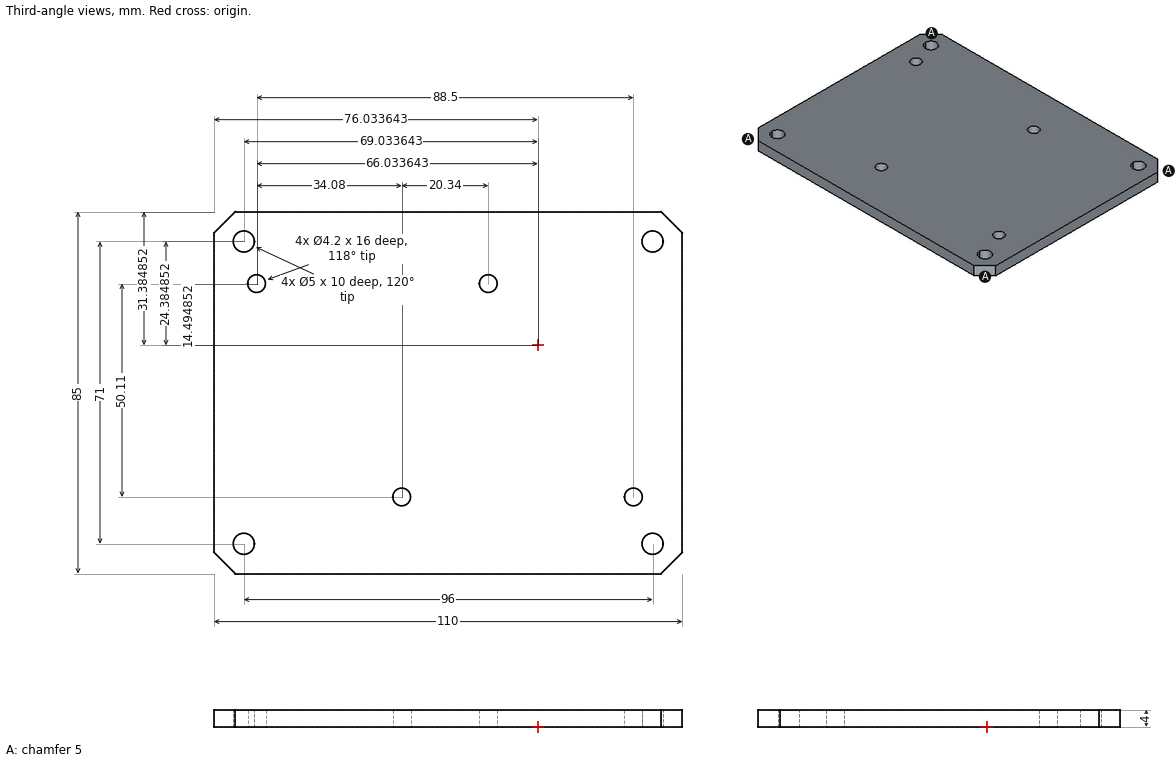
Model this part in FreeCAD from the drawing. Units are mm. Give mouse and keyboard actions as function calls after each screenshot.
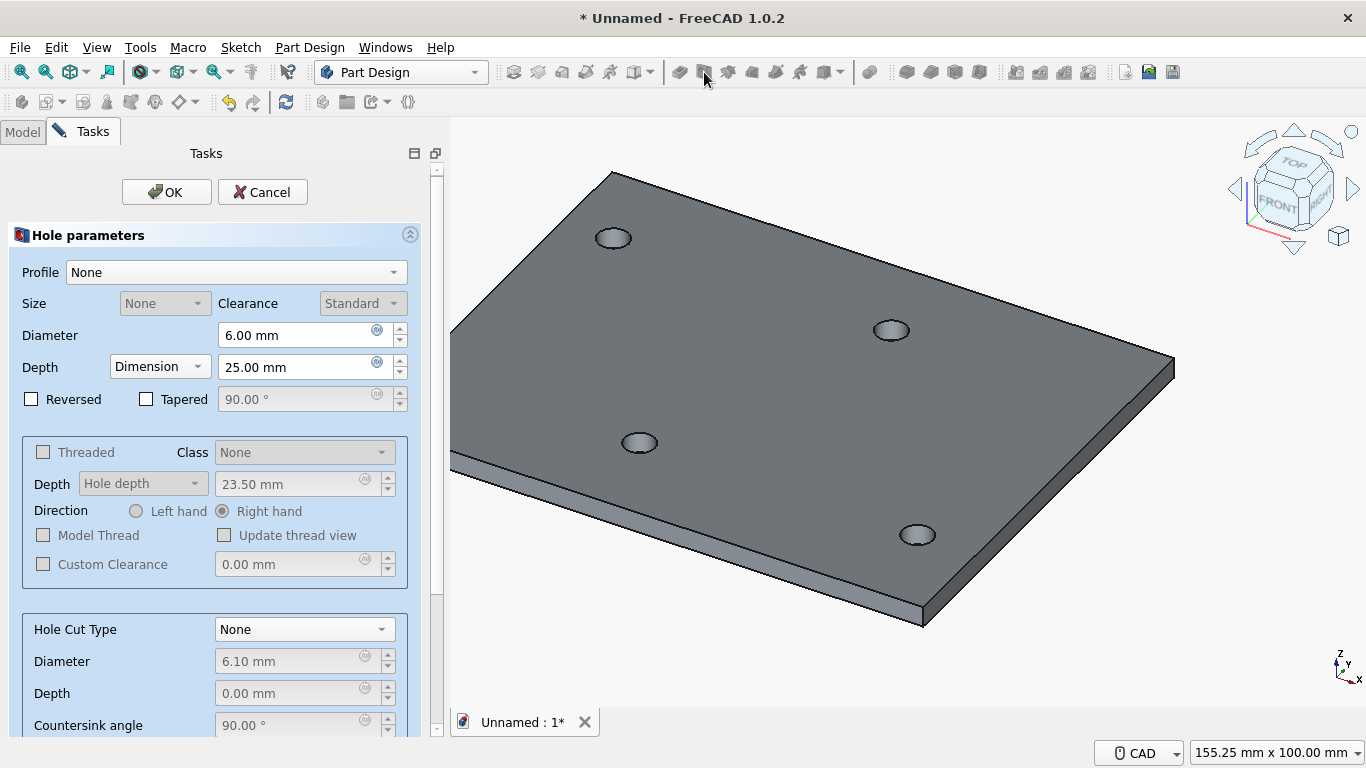
triple_click(305, 335)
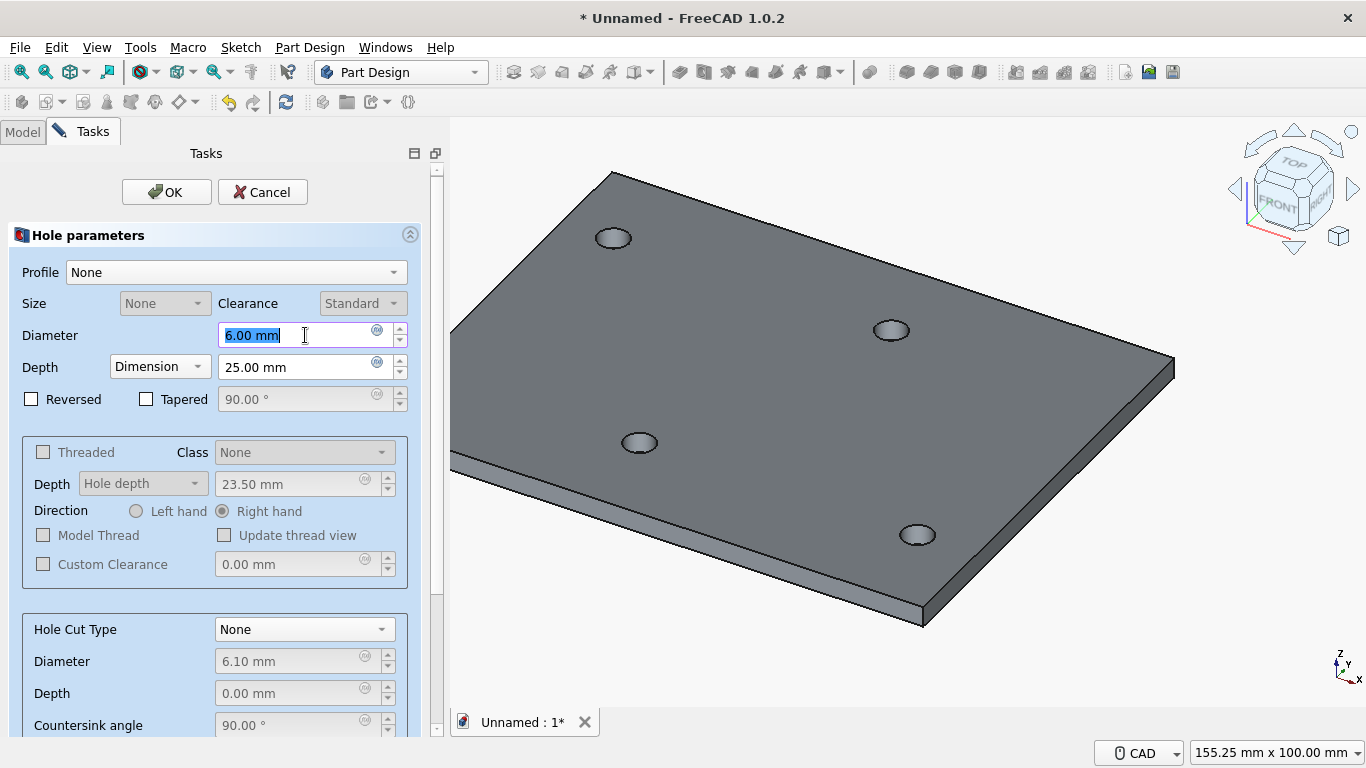
text(4.2)
key(Tab)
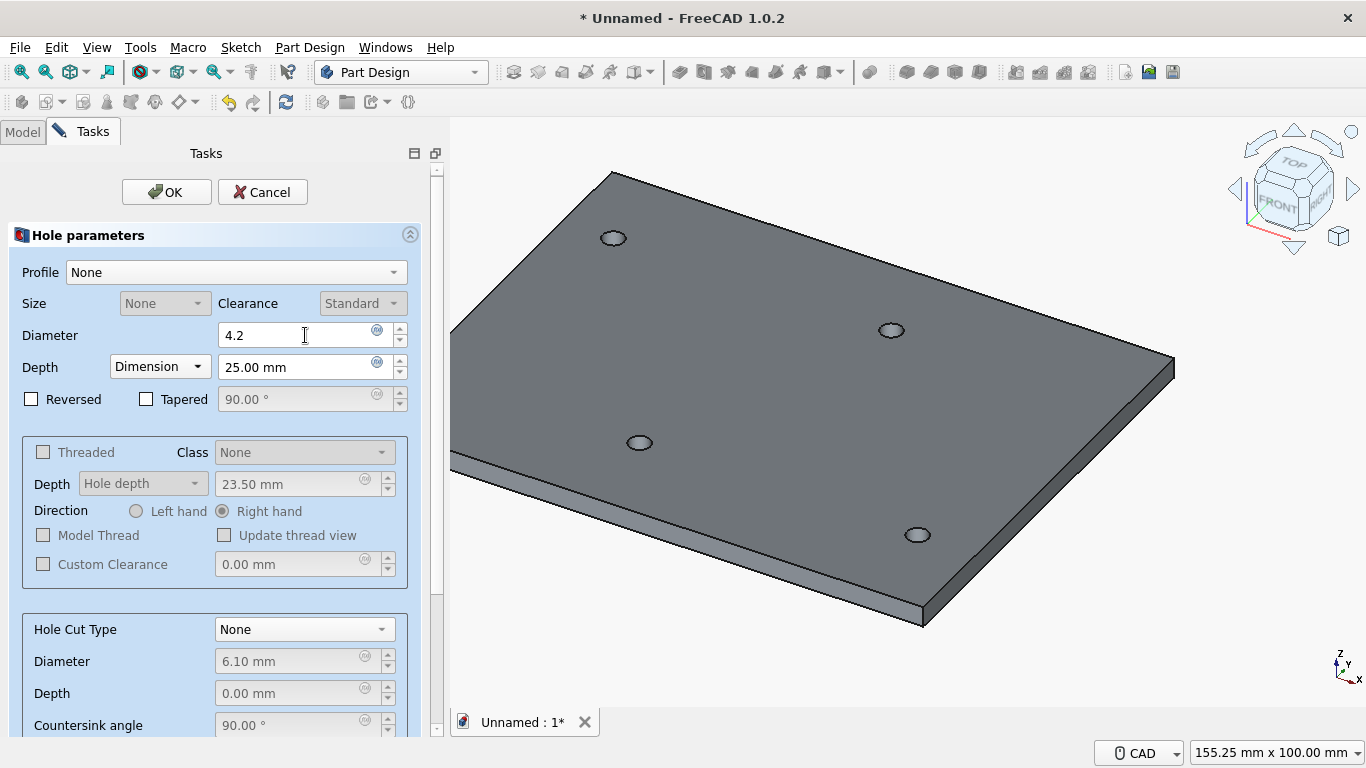
triple_click(305, 367)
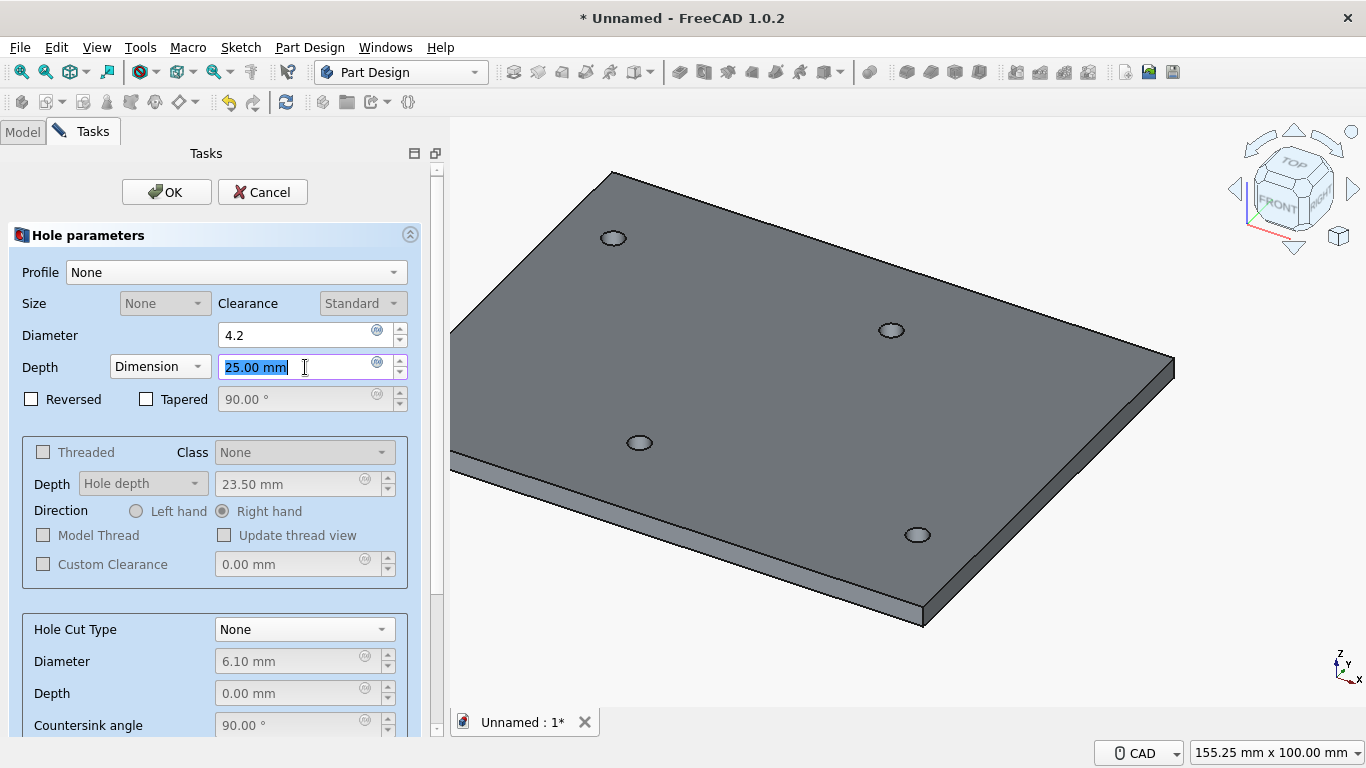
text(16)
key(Tab)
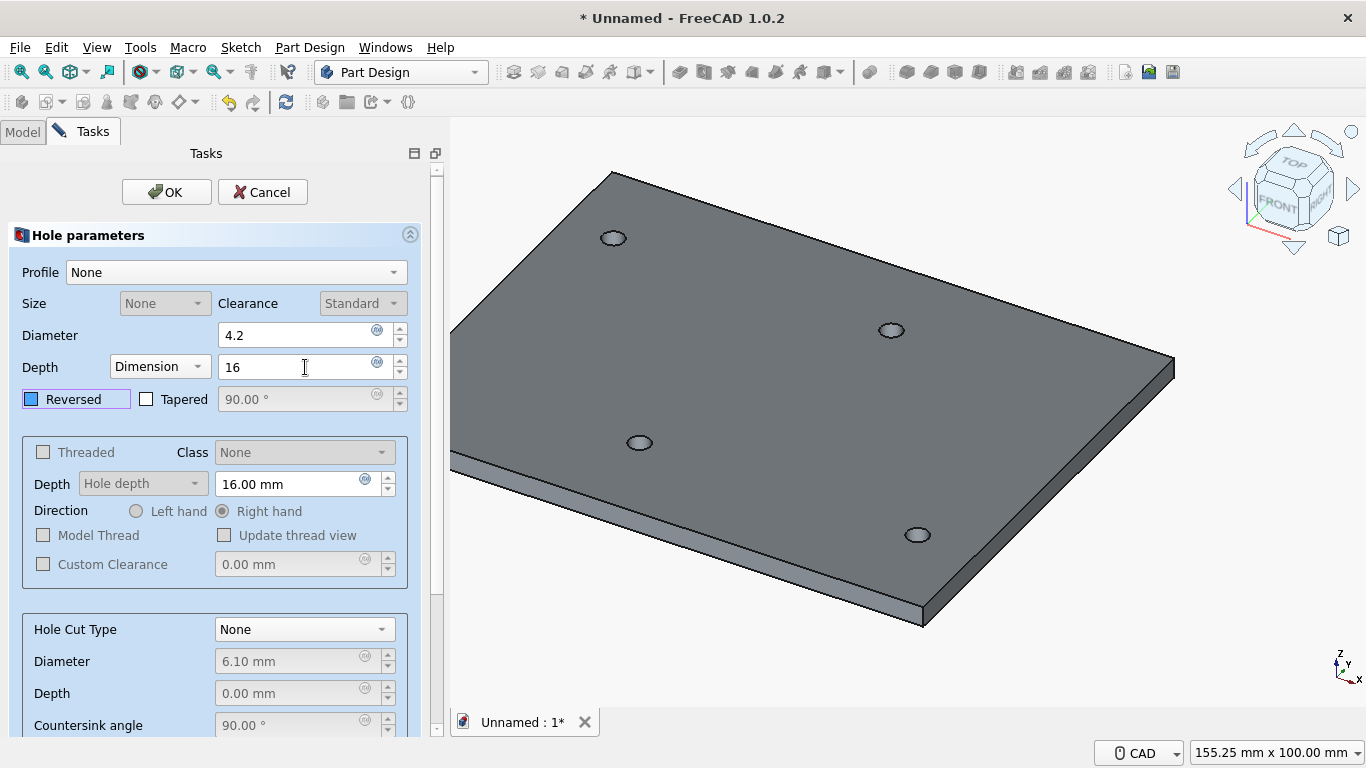
click(167, 192)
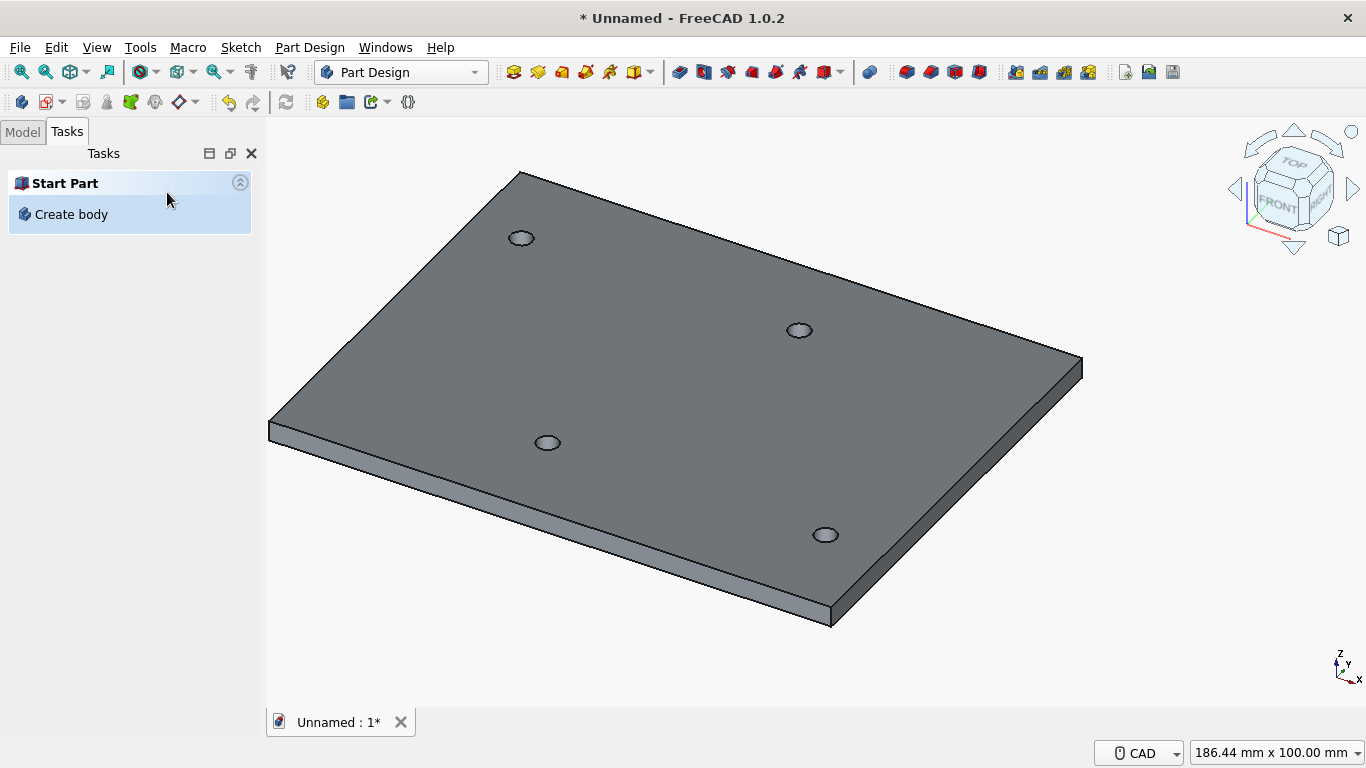
click(831, 616)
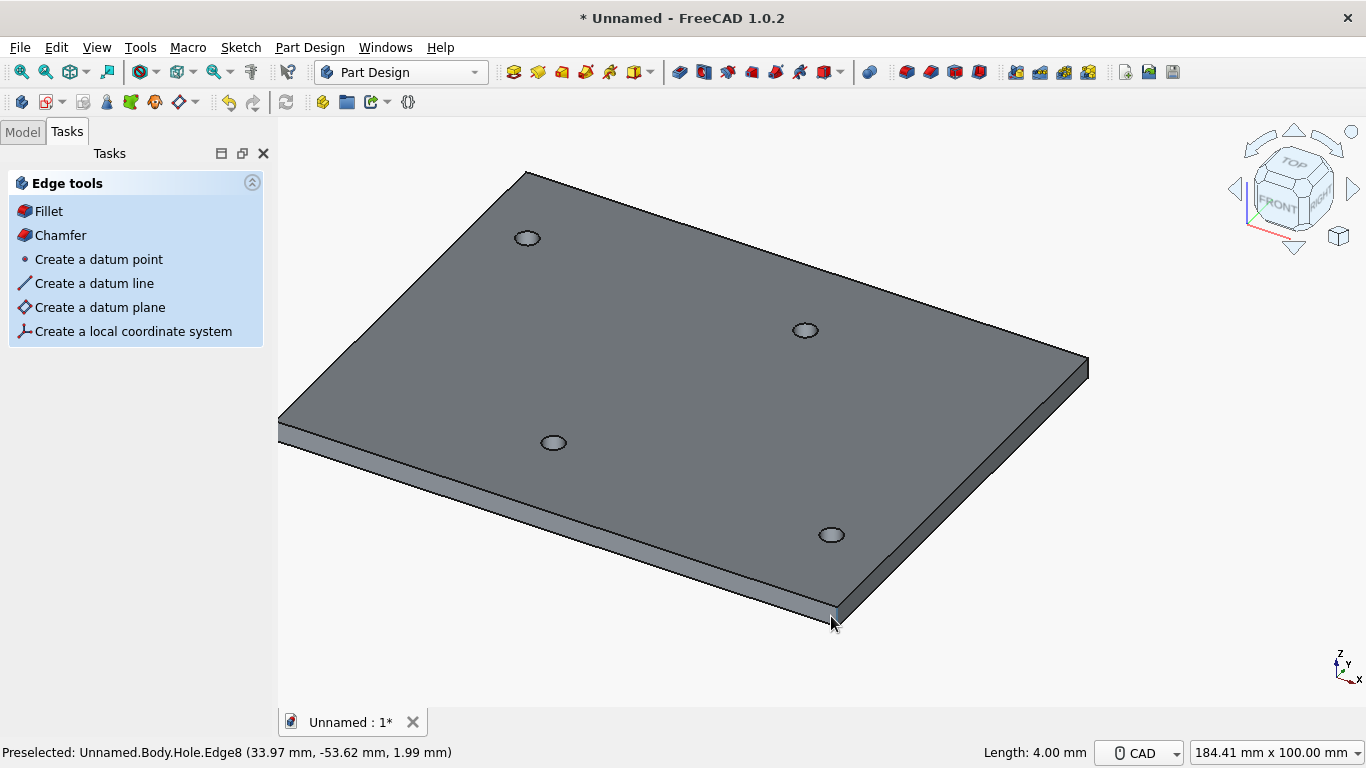
key(0)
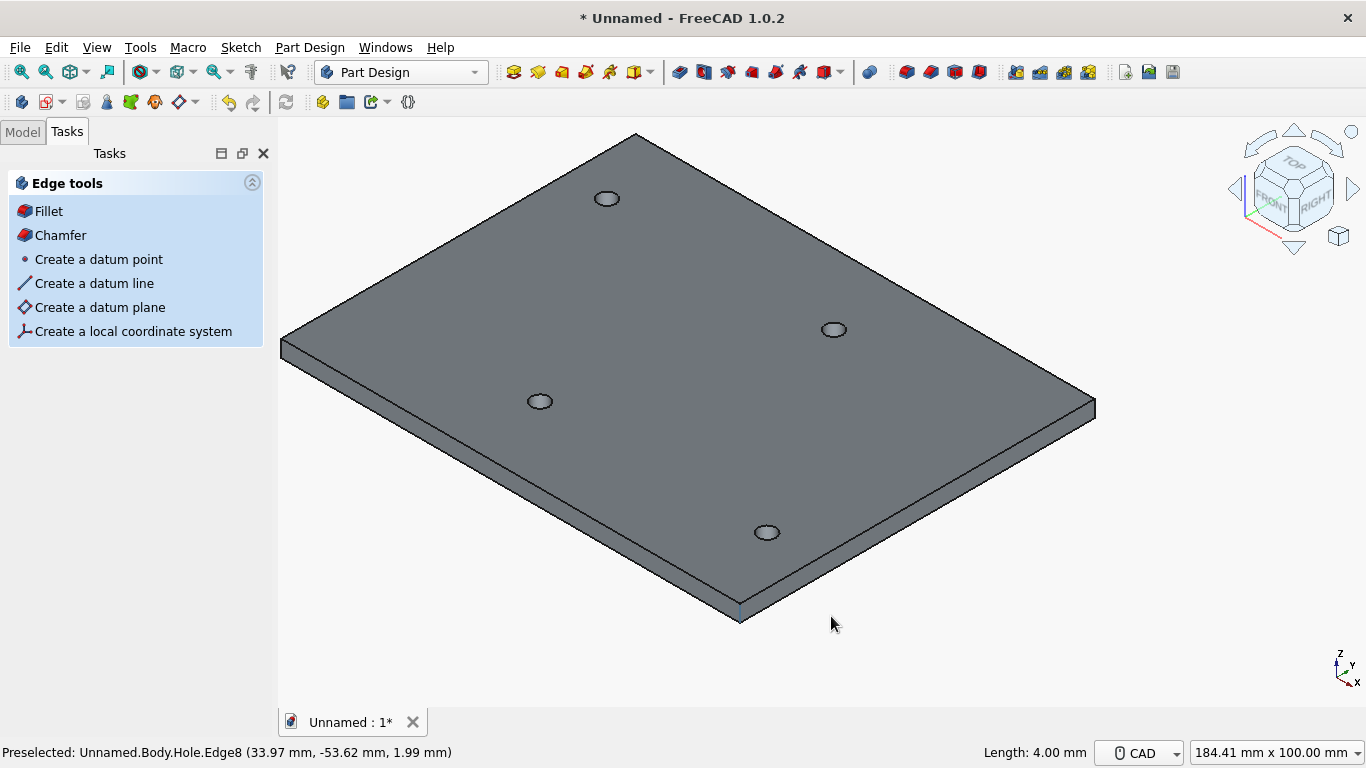
key(2)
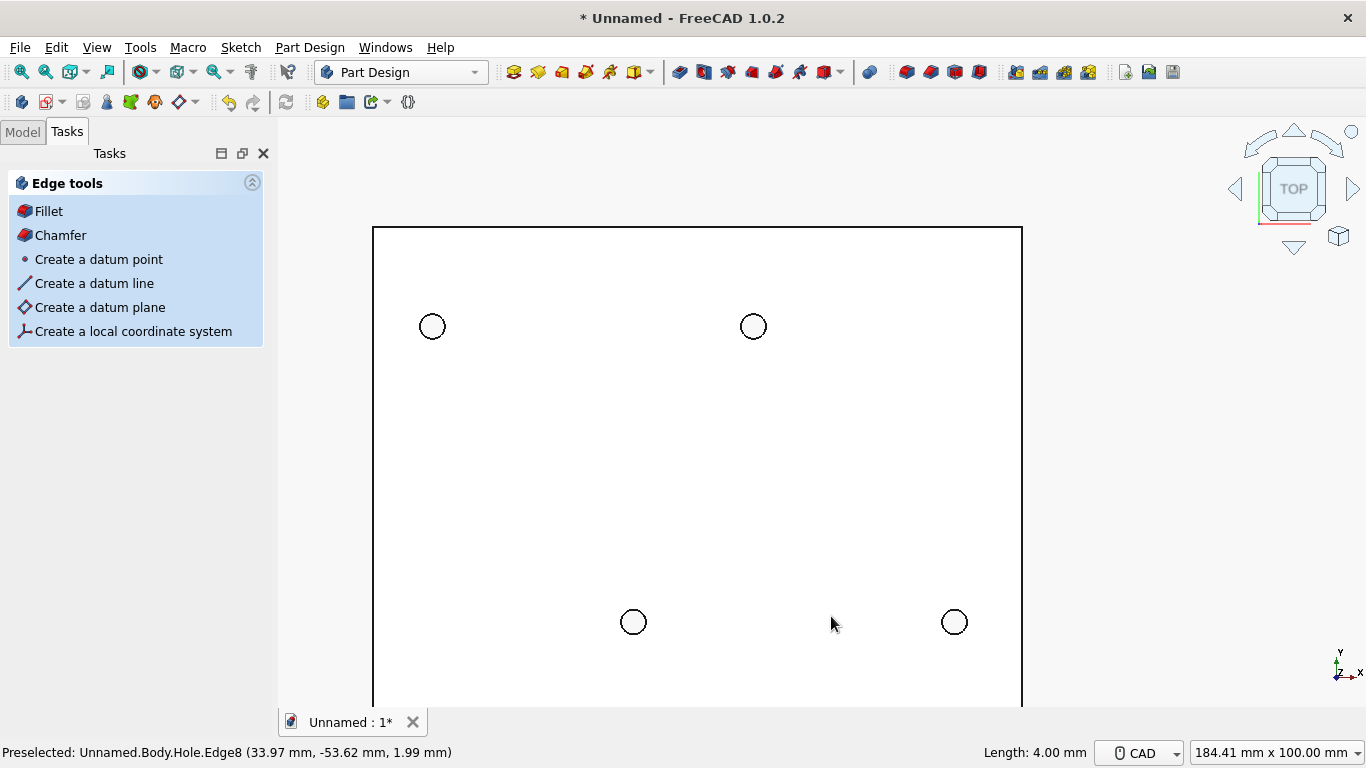
click(22, 72)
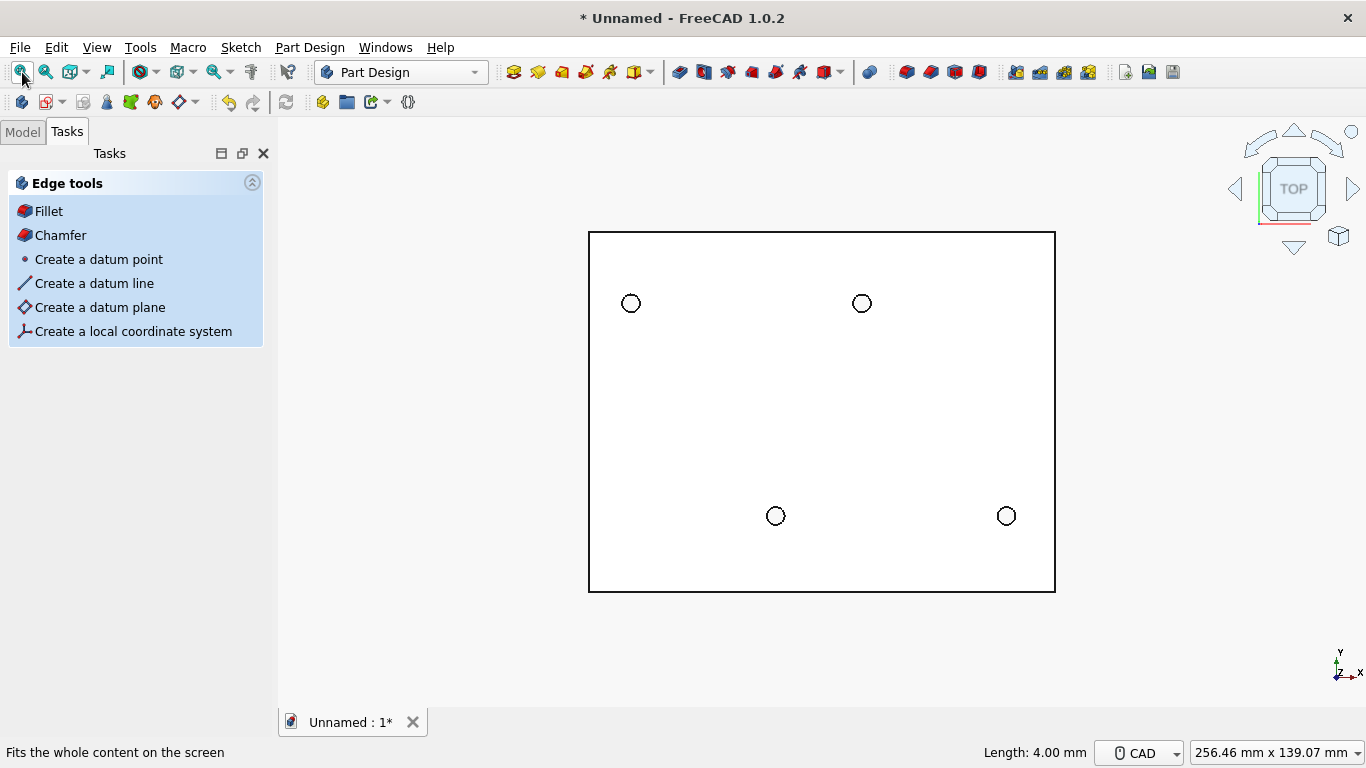
scroll(589, 231, up, 5)